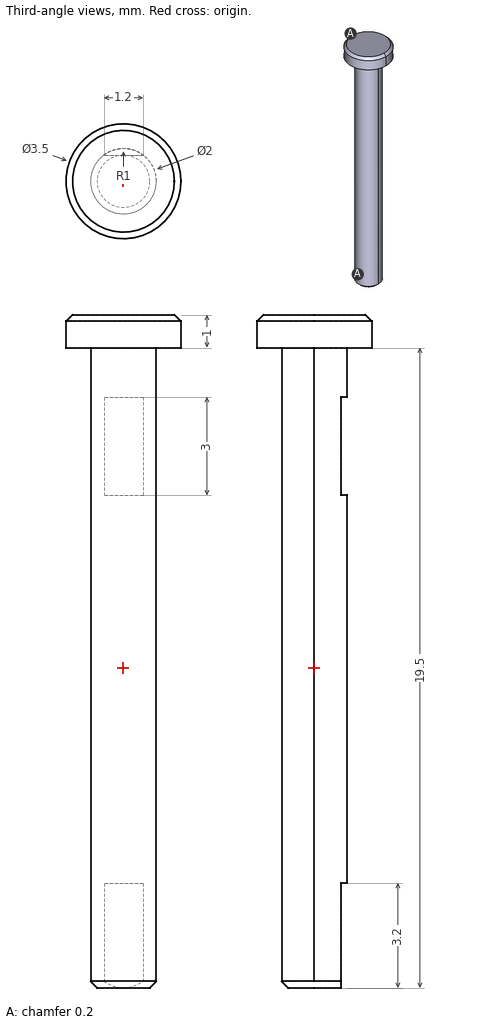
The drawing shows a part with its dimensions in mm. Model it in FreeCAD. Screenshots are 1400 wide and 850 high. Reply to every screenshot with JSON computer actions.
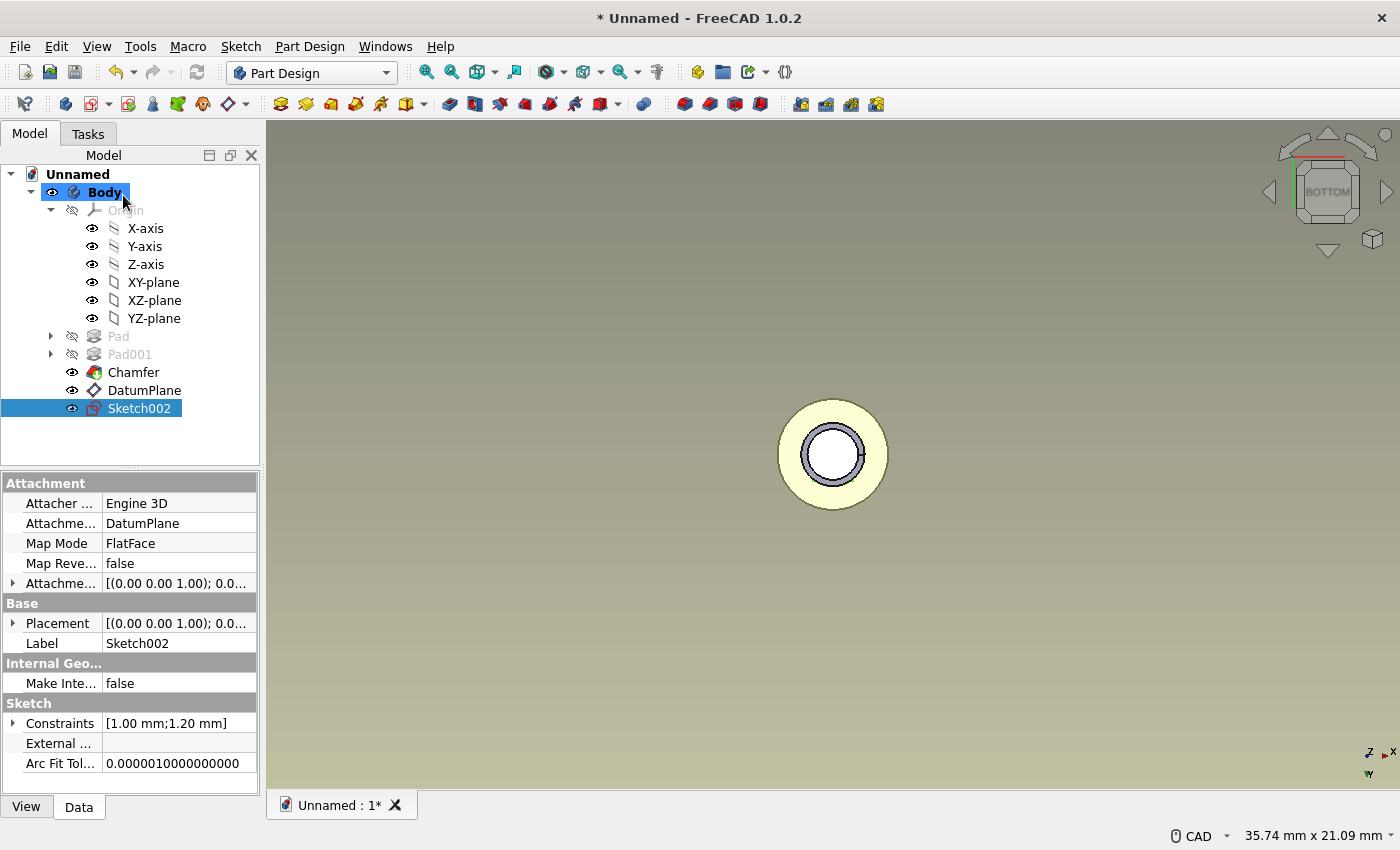
{"action": "left_click", "coordinate": [450, 104]}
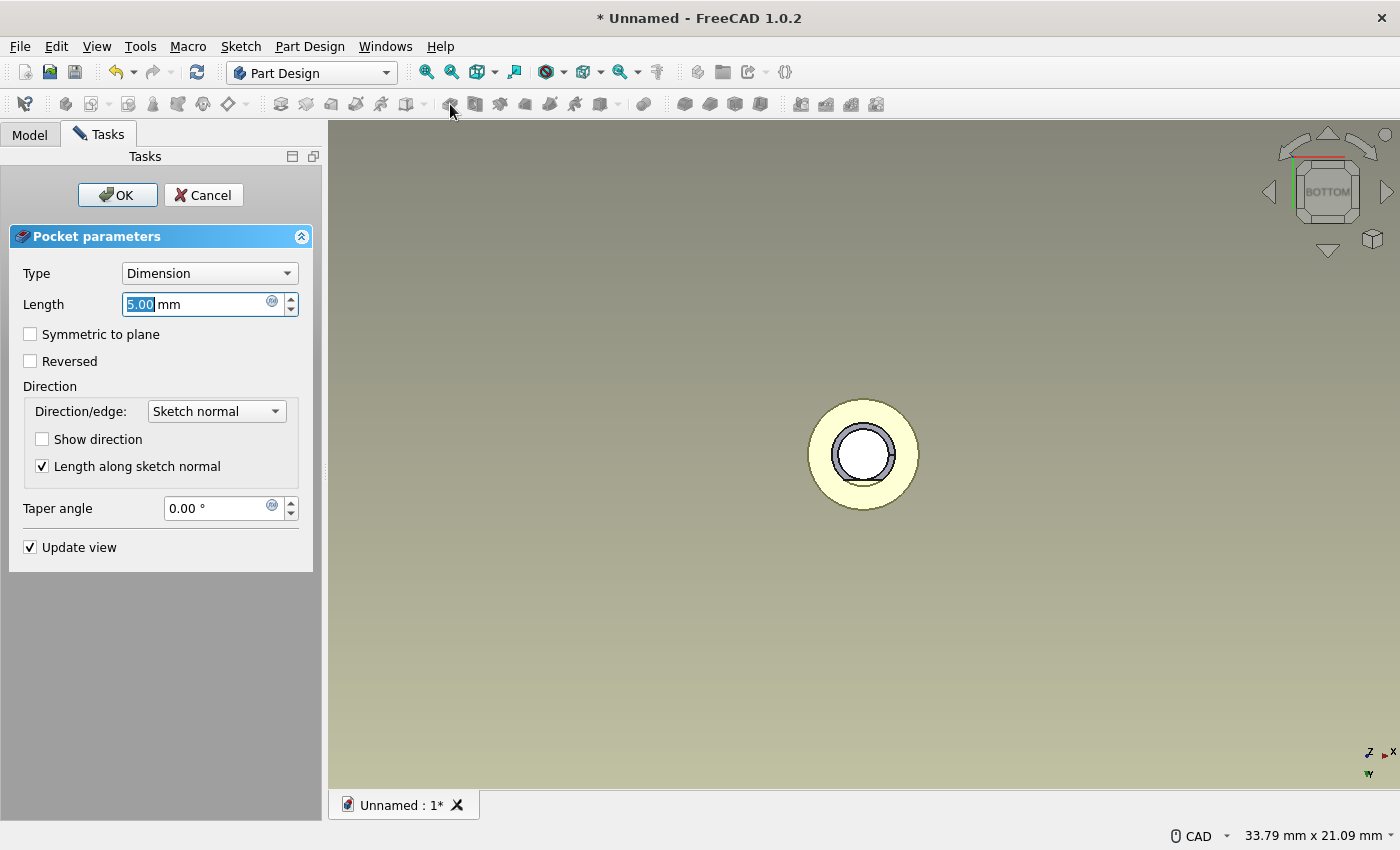
{"action": "type", "text": "3.2"}
{"action": "key", "text": "Tab"}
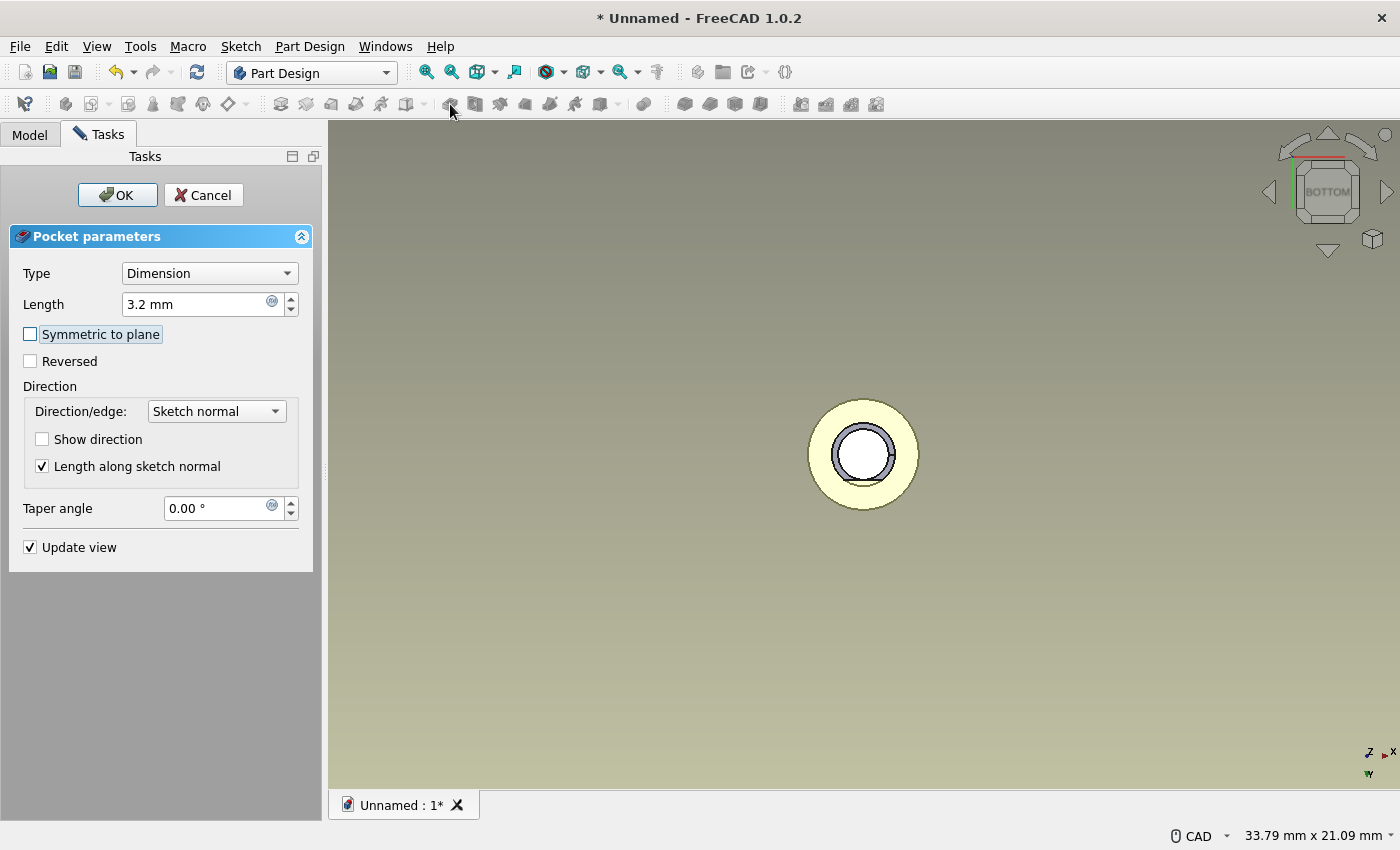
{"action": "left_click", "coordinate": [118, 195]}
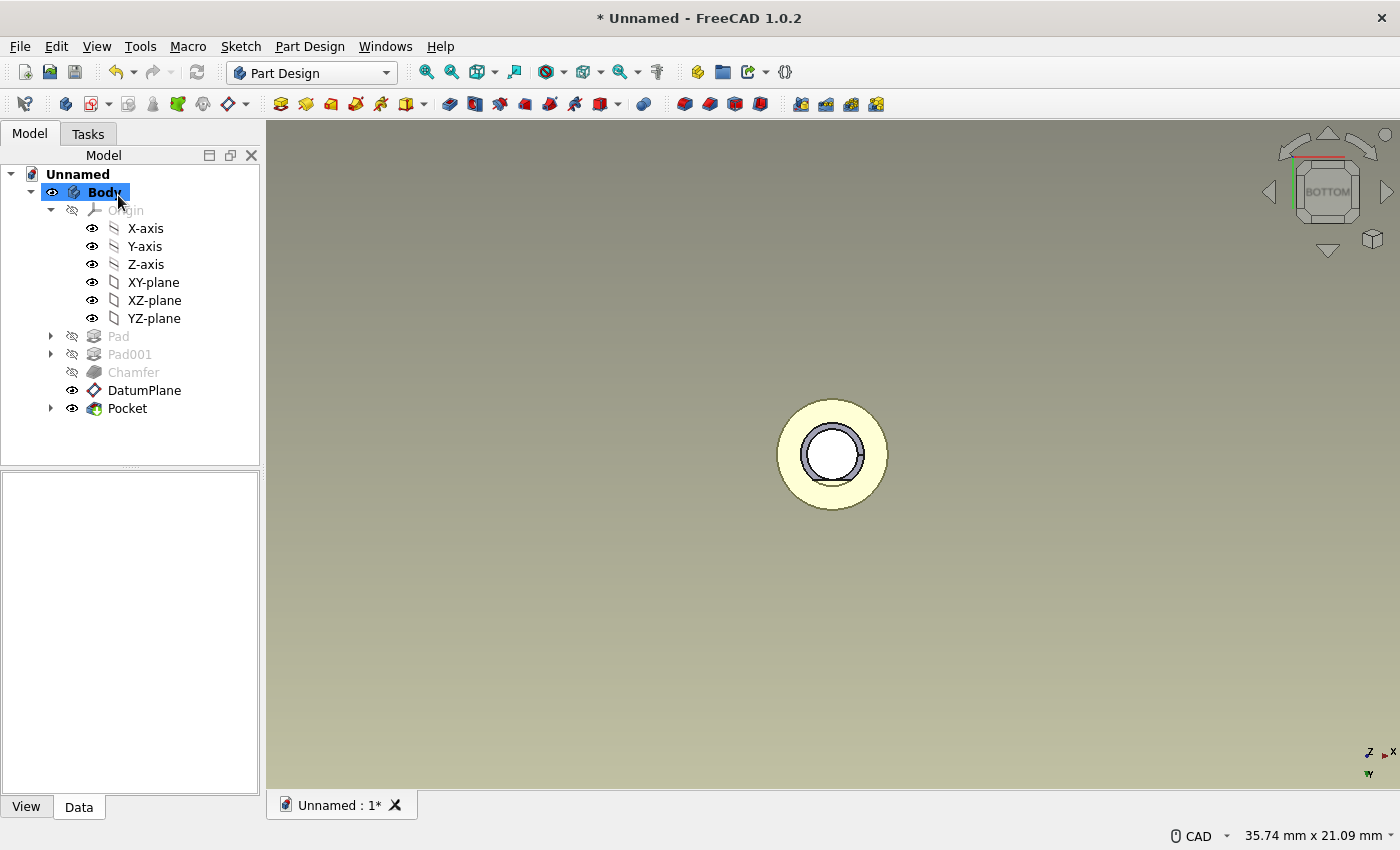
{"action": "left_click", "coordinate": [117, 390]}
{"action": "key", "text": "space"}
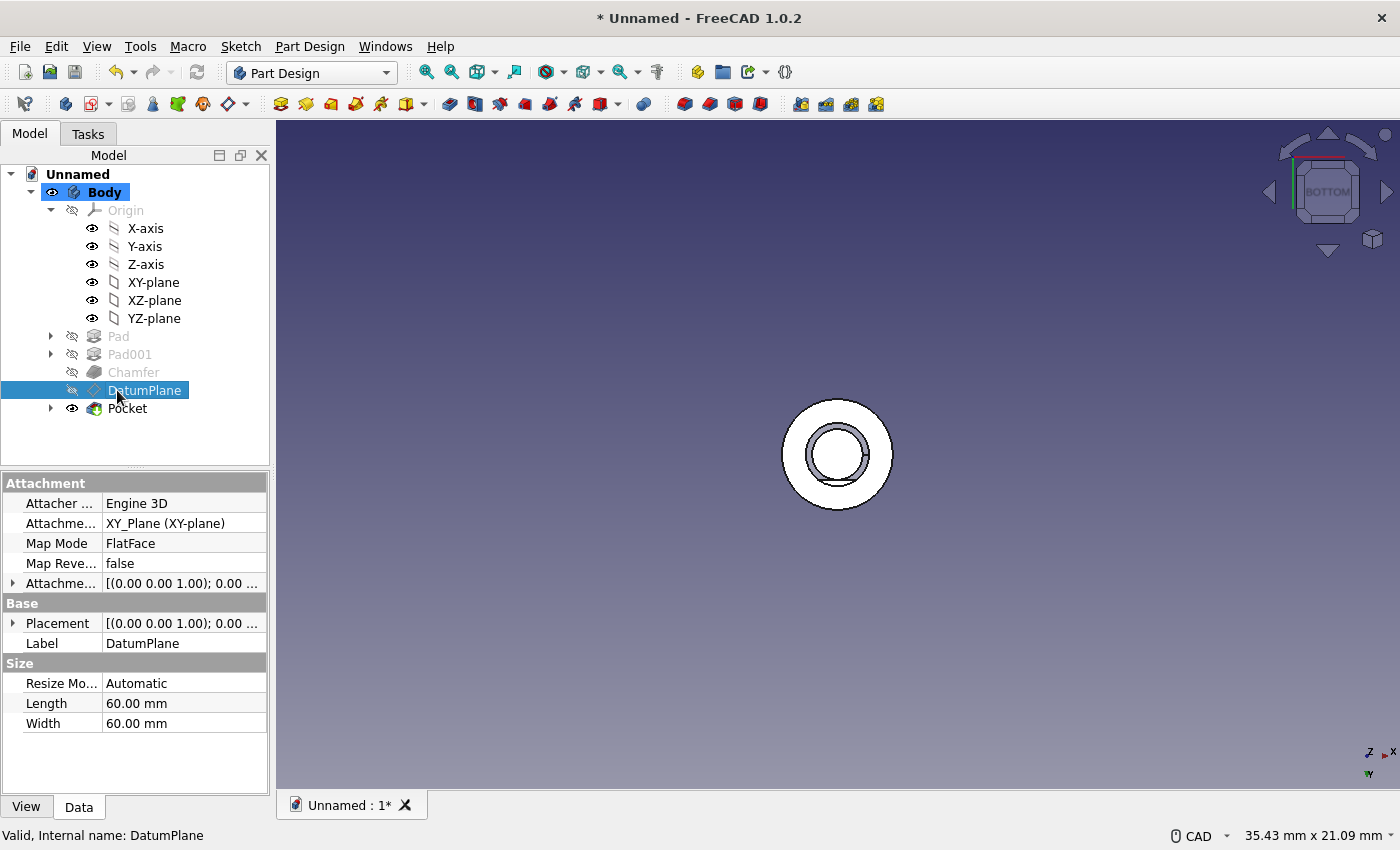
{"action": "left_click", "coordinate": [427, 72]}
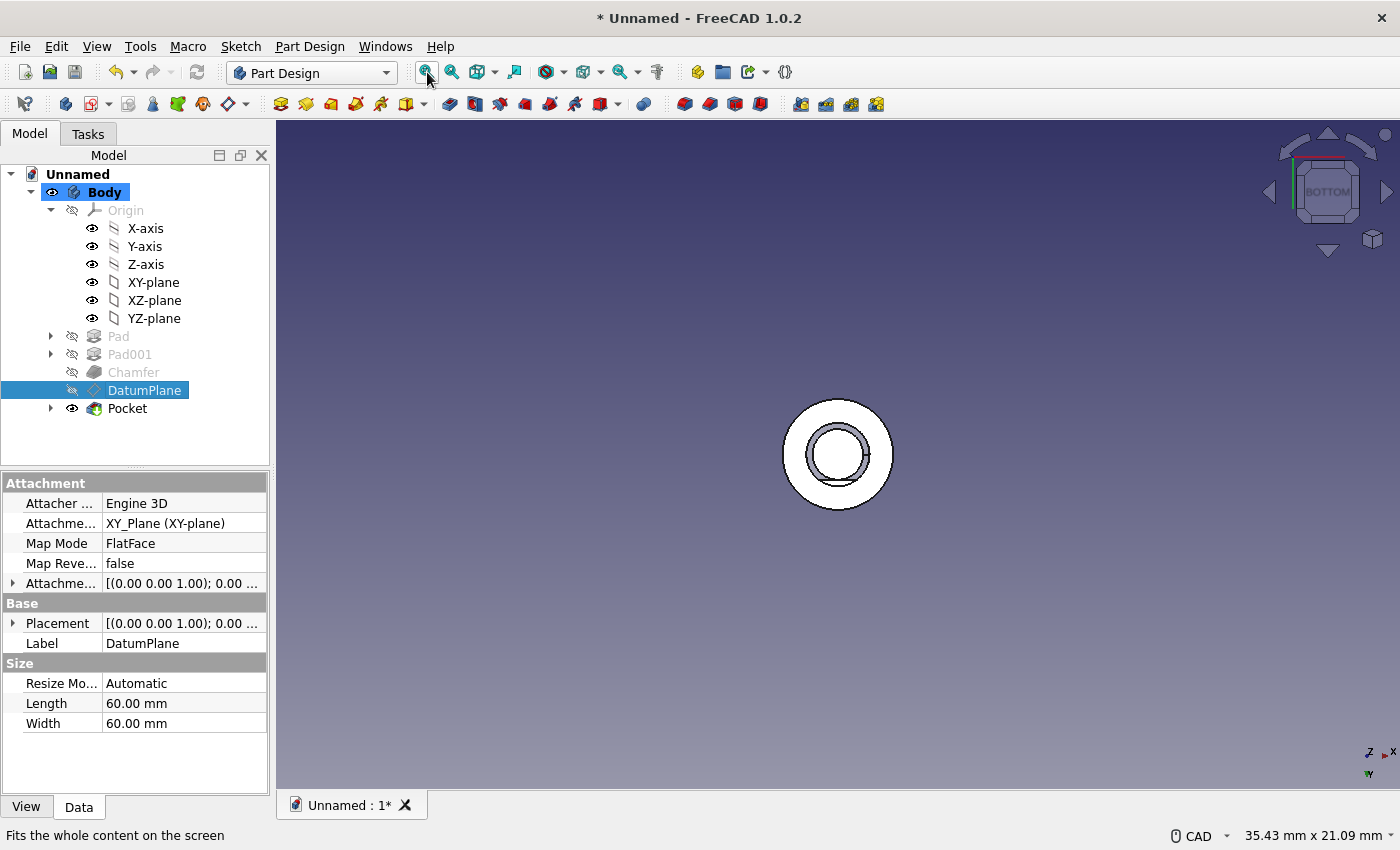
{"action": "left_click", "coordinate": [137, 282]}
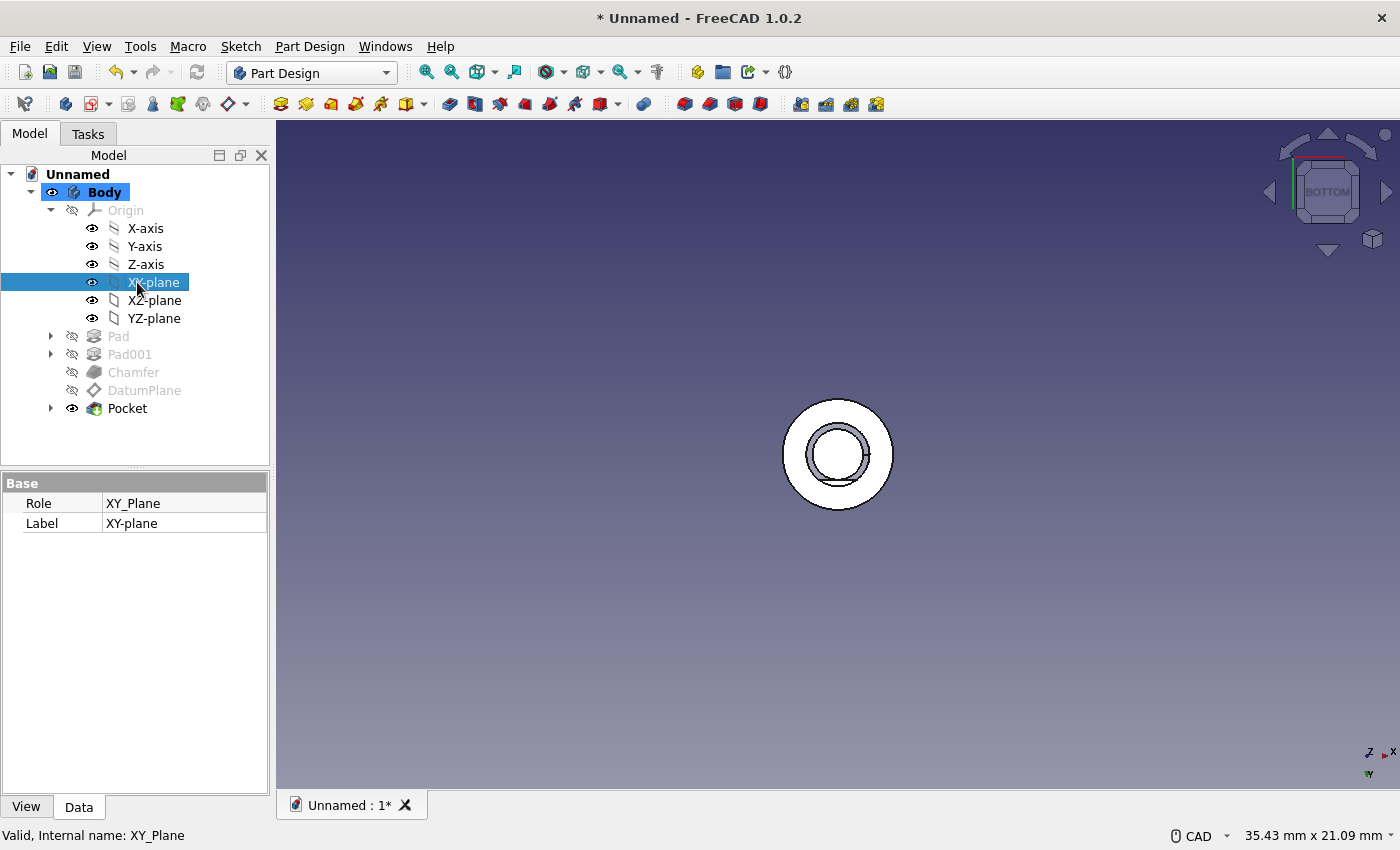
{"action": "left_click", "coordinate": [228, 104]}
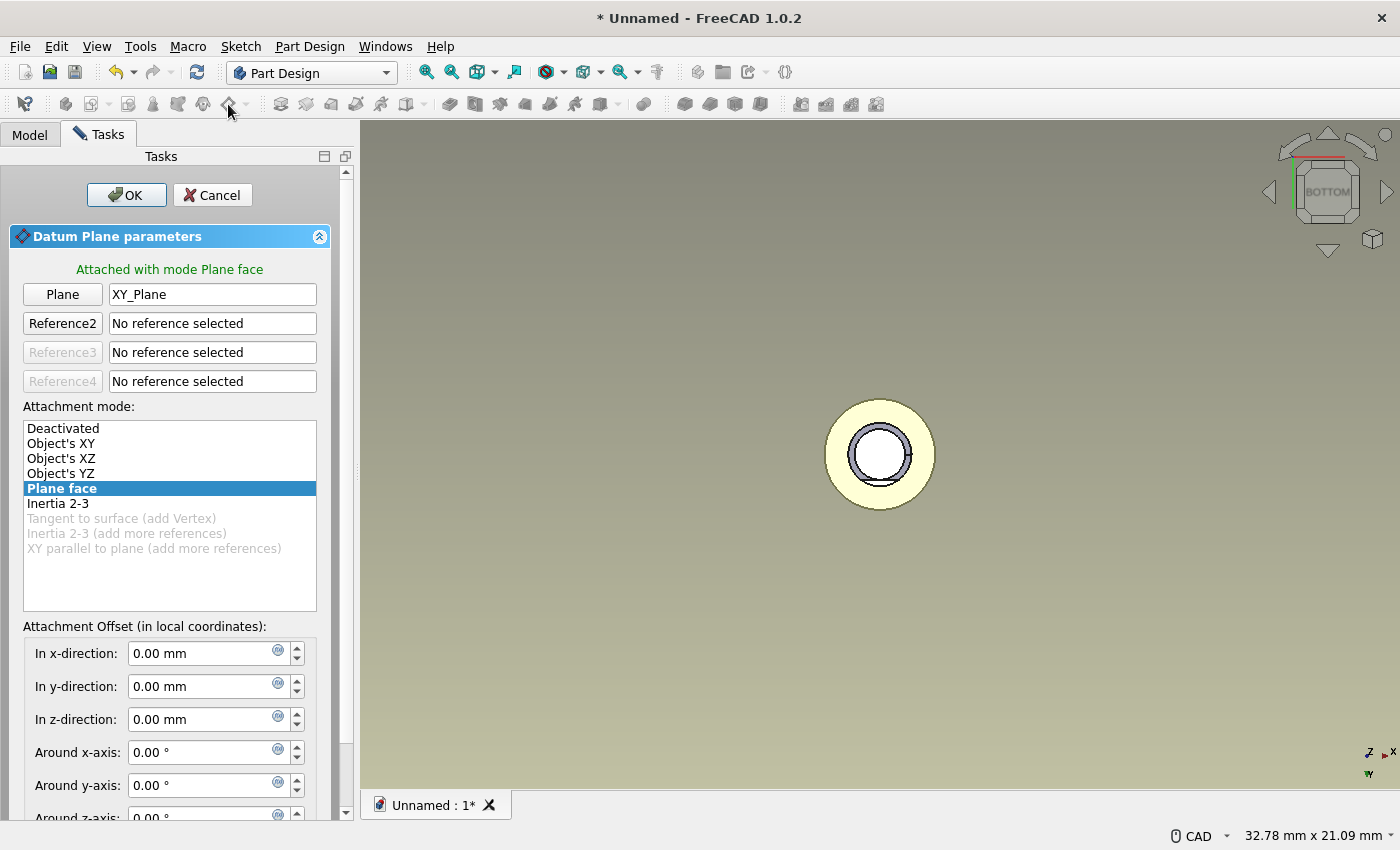
{"action": "triple_click", "coordinate": [210, 720]}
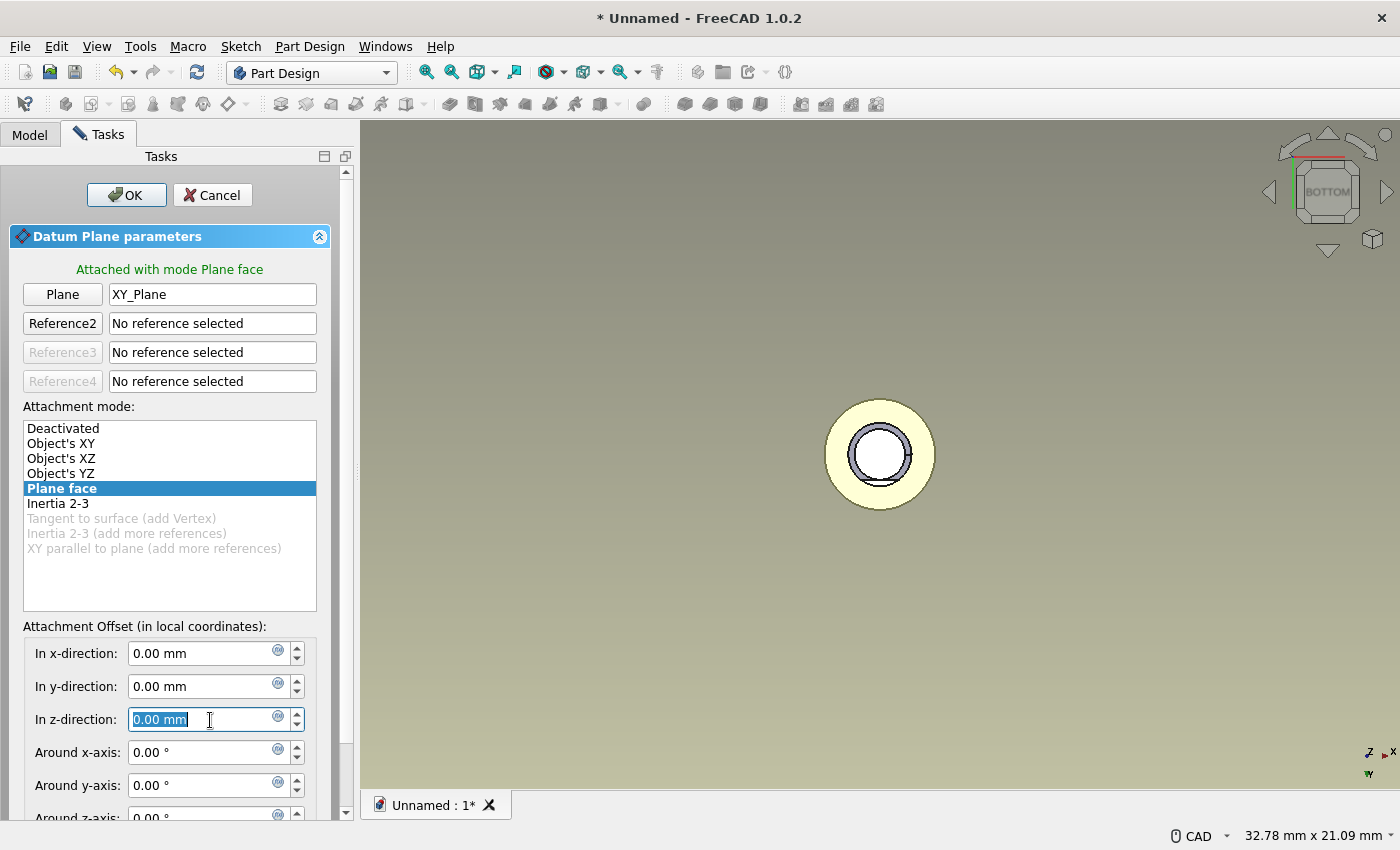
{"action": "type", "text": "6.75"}
{"action": "key", "text": "Tab"}